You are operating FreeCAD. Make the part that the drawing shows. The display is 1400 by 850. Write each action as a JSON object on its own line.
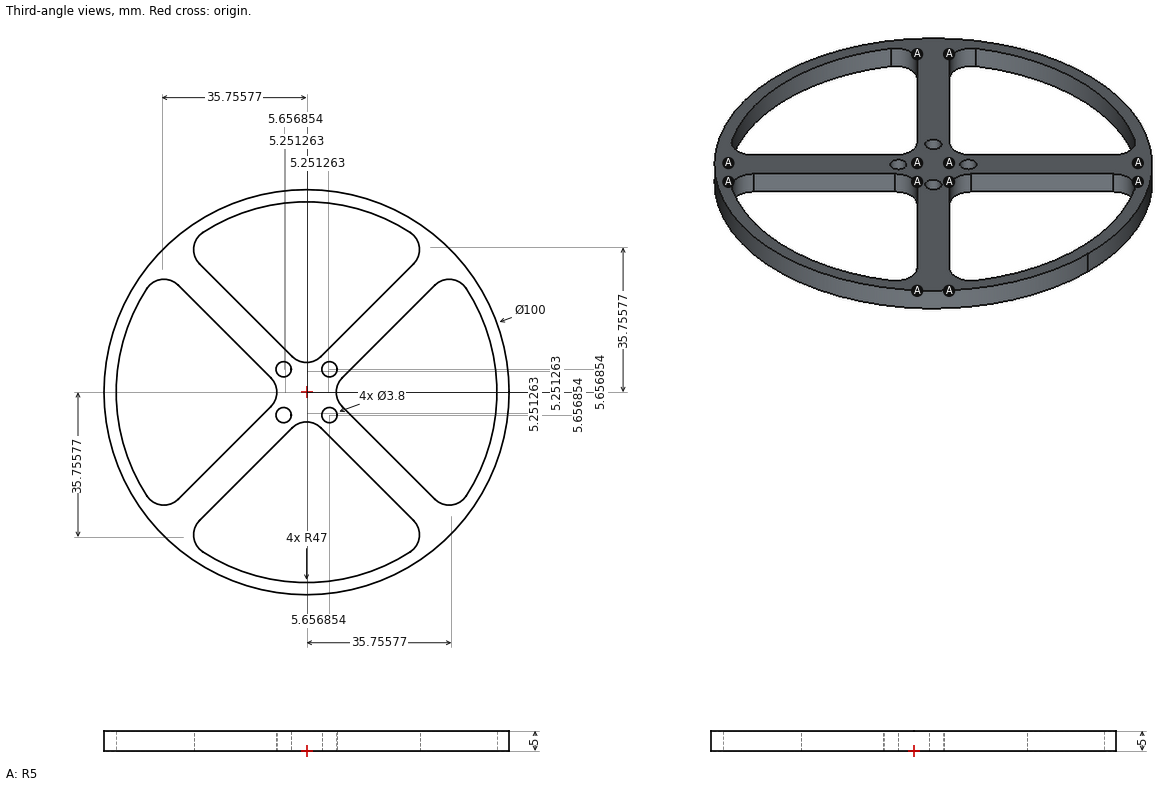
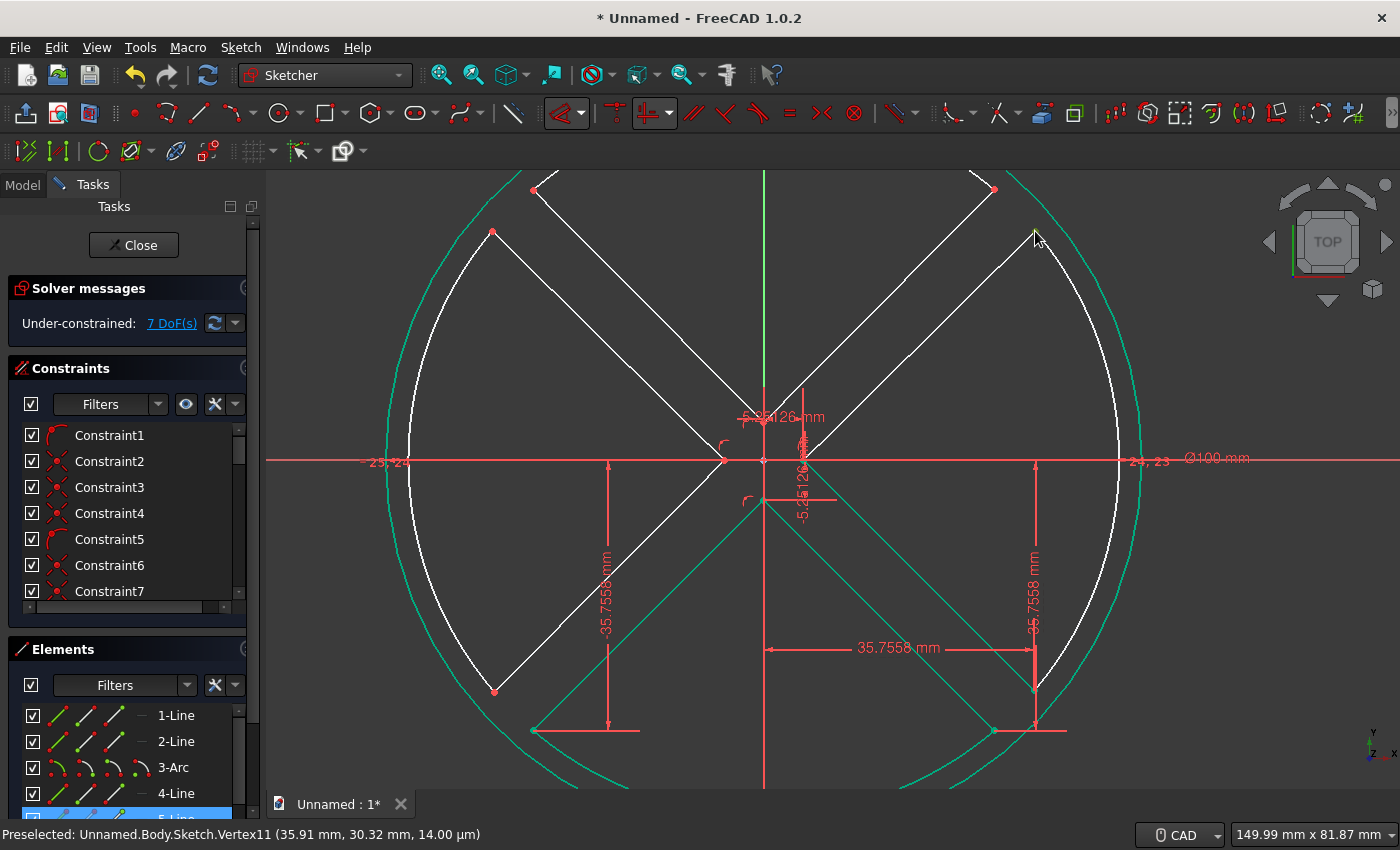
{"action": "key", "text": "l"}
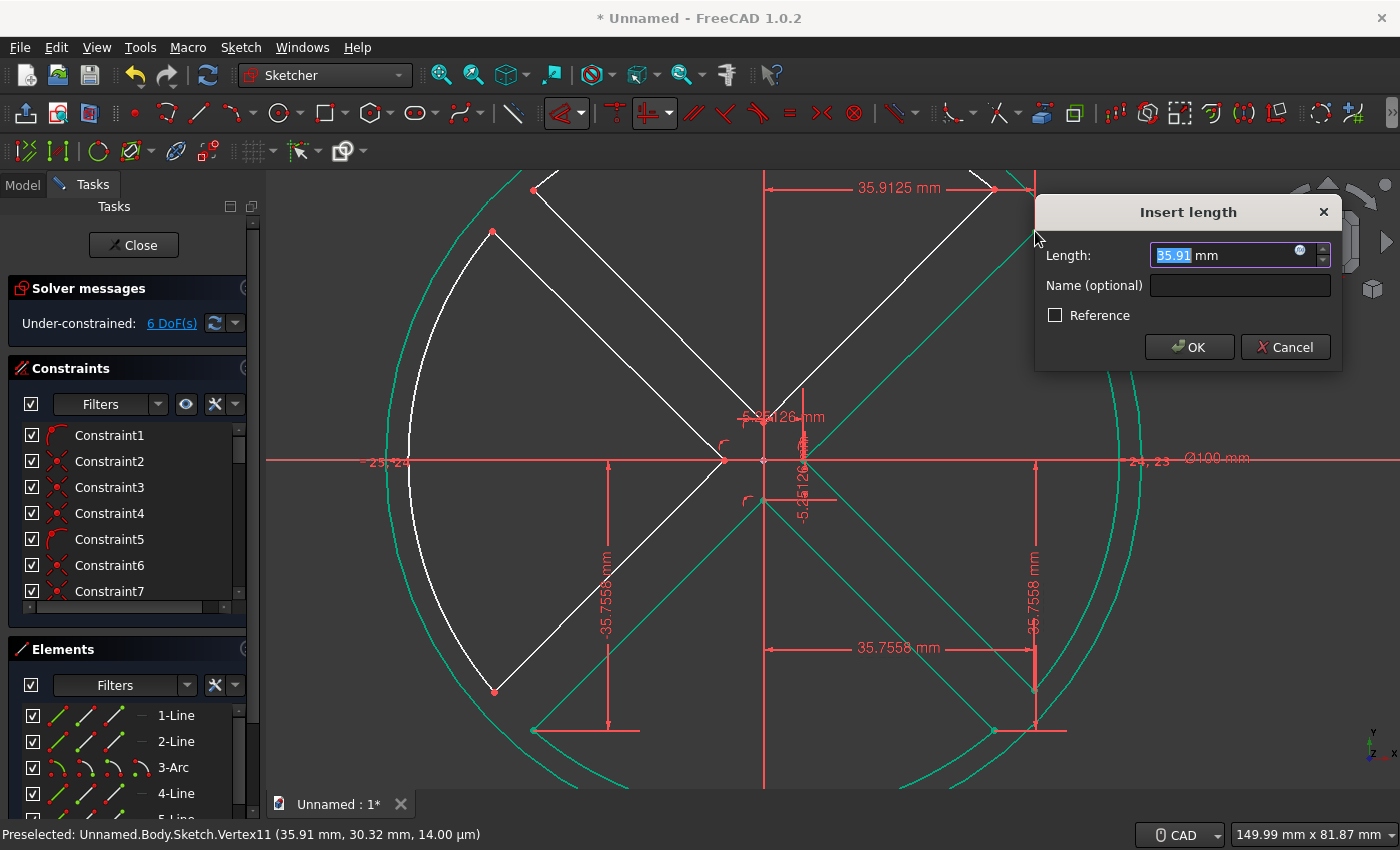
{"action": "type", "text": "35.75577"}
{"action": "key", "text": "Return"}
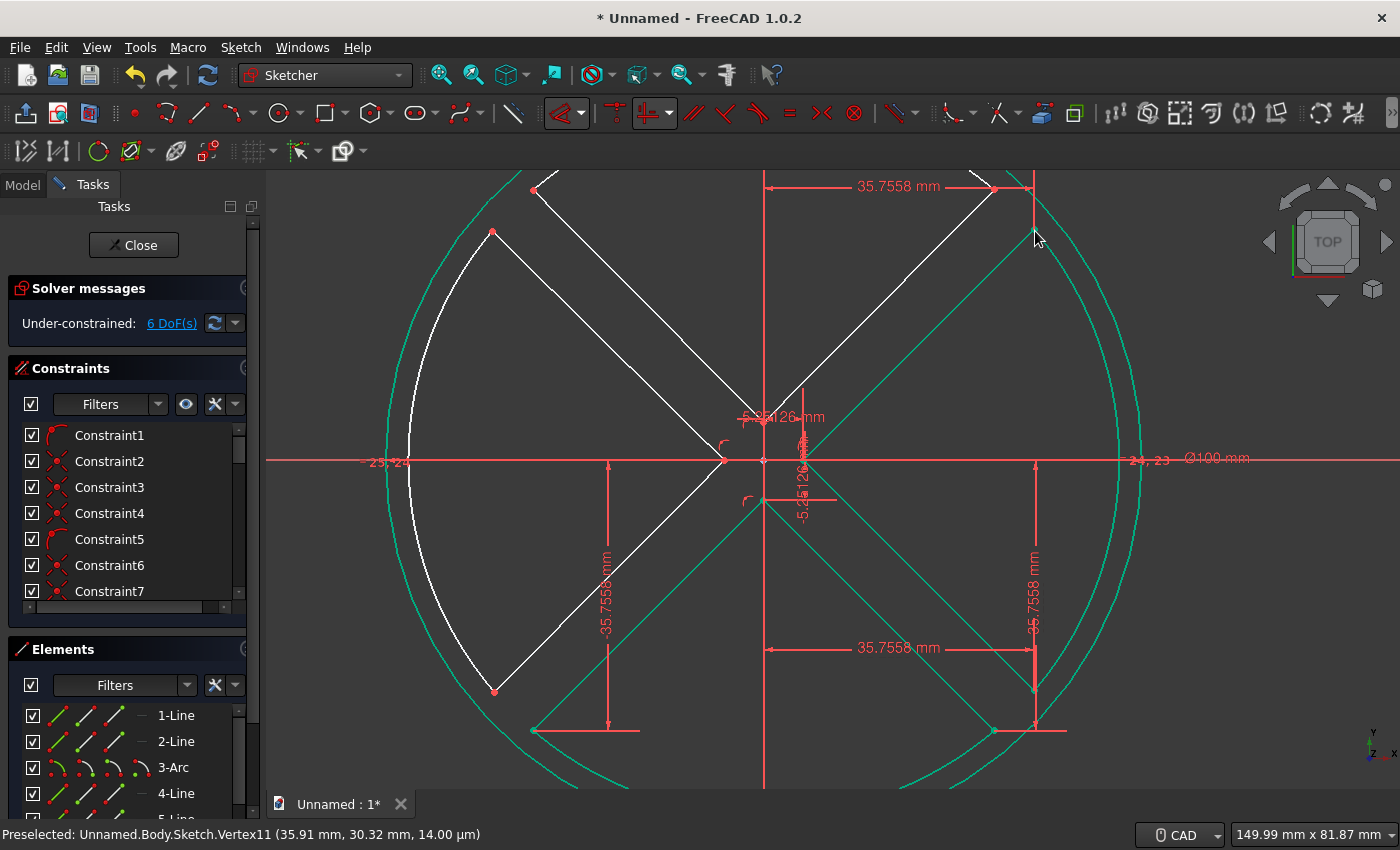
{"action": "left_click", "coordinate": [492, 231]}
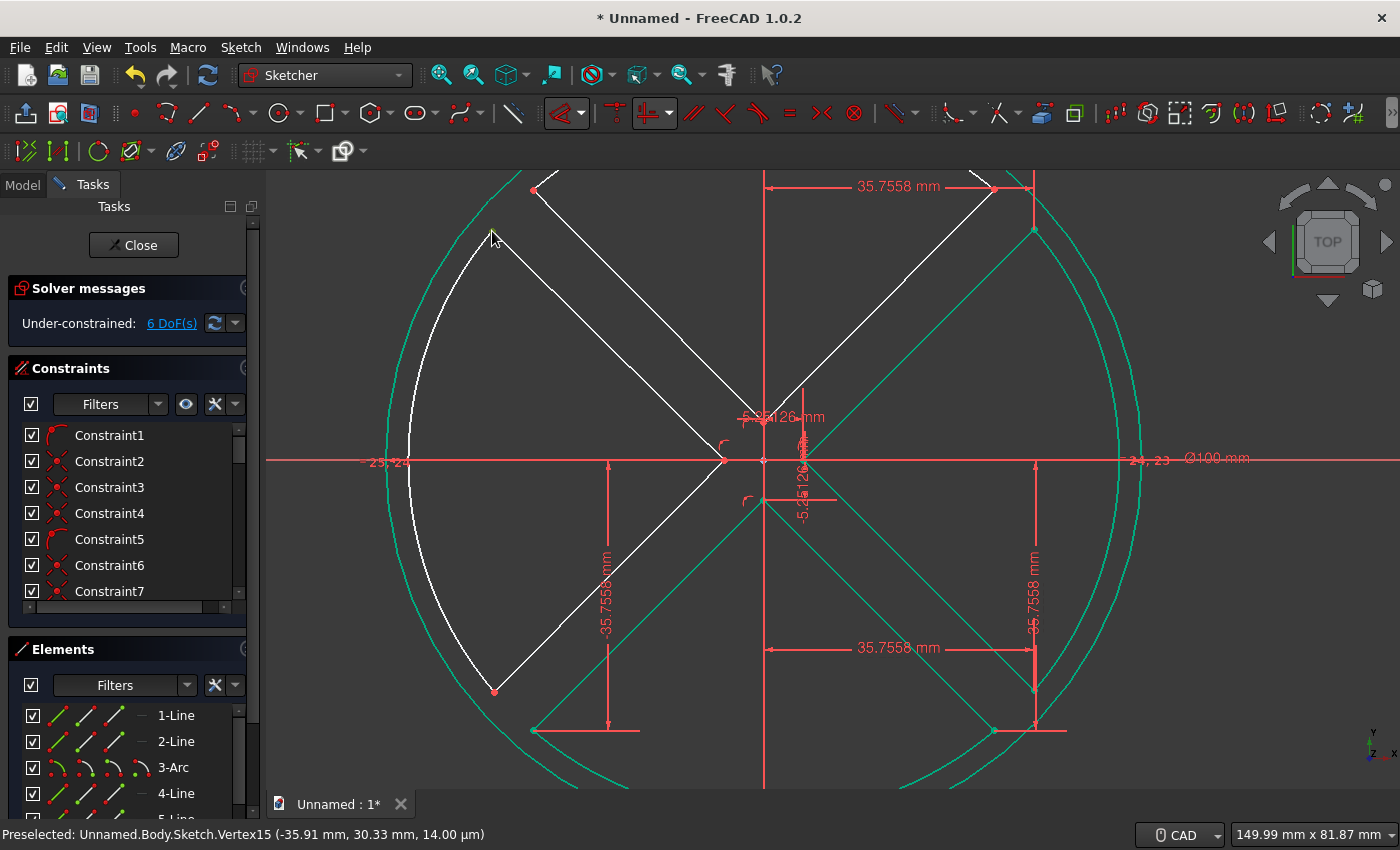
{"action": "key", "text": "l"}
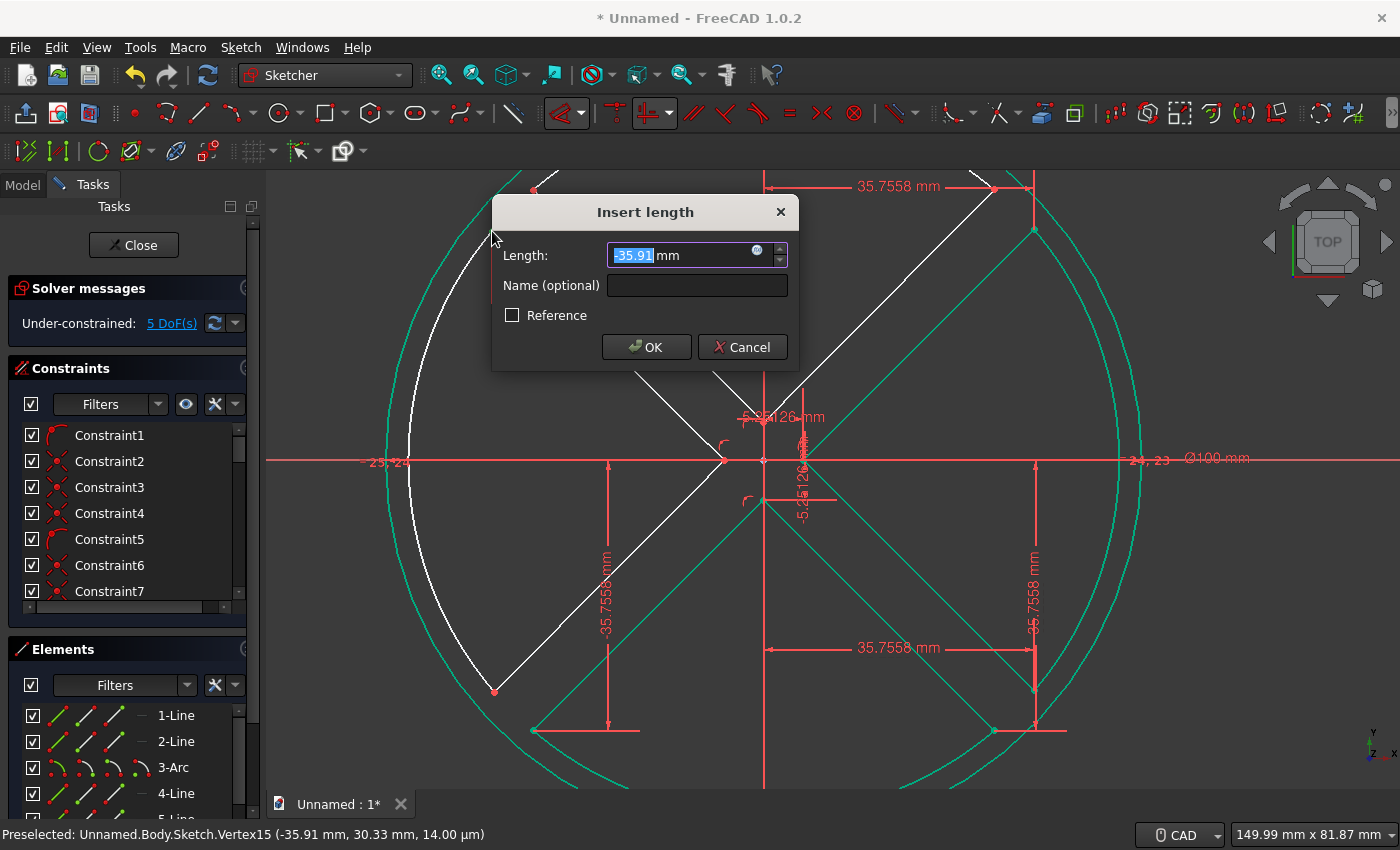
{"action": "type", "text": "-35.75577"}
{"action": "key", "text": "Return"}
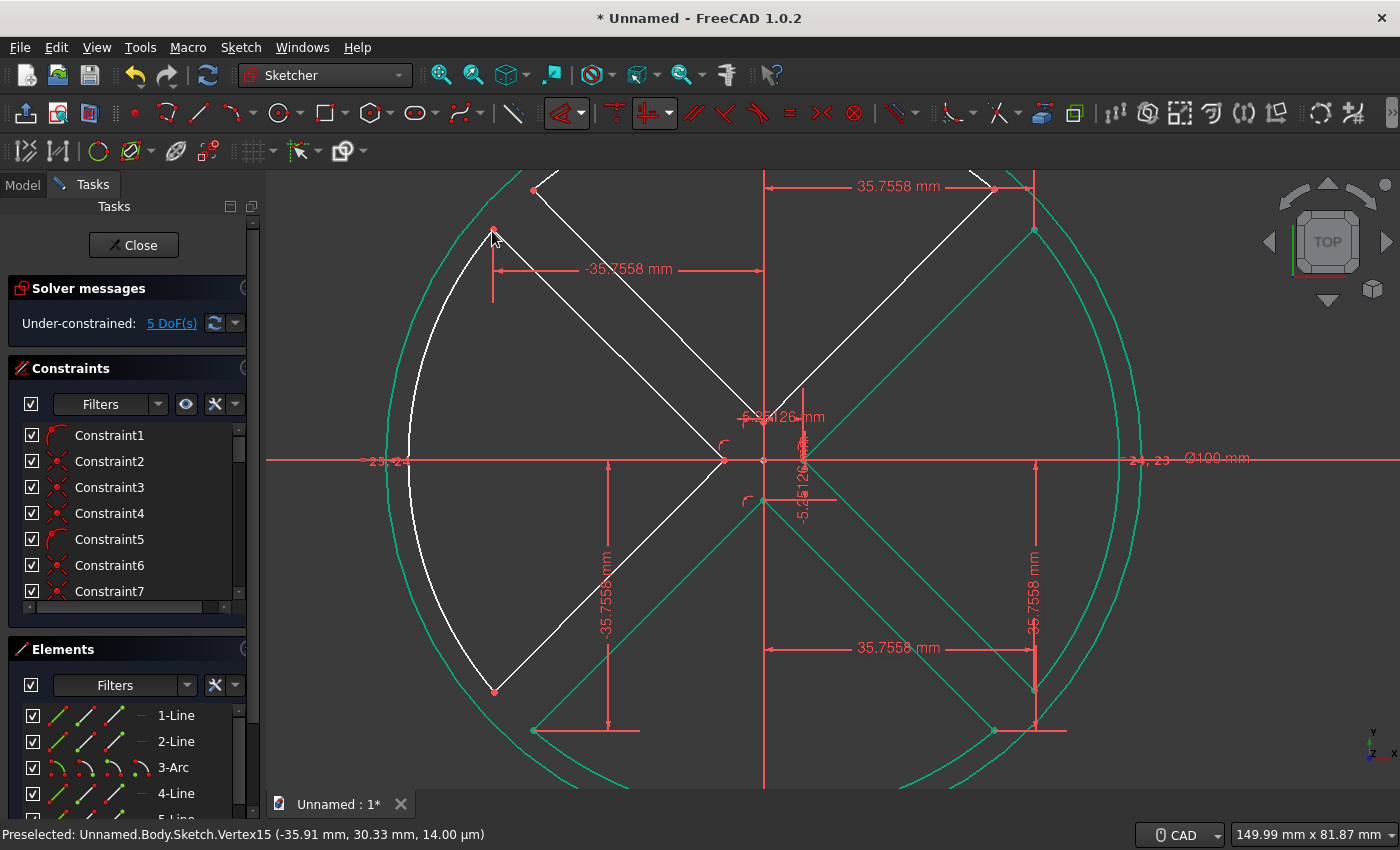
{"action": "left_click", "coordinate": [725, 460]}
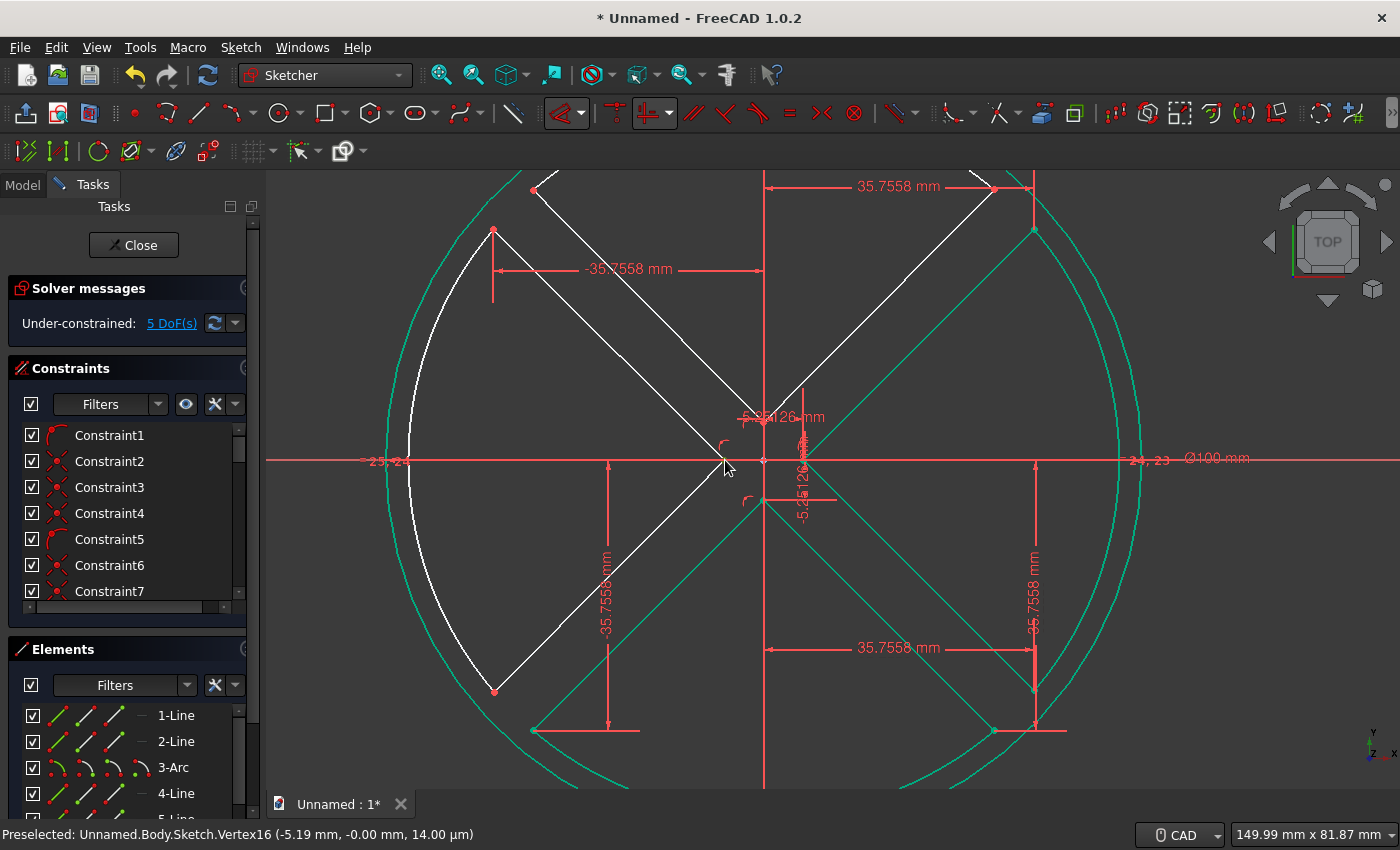
{"action": "key", "text": "l"}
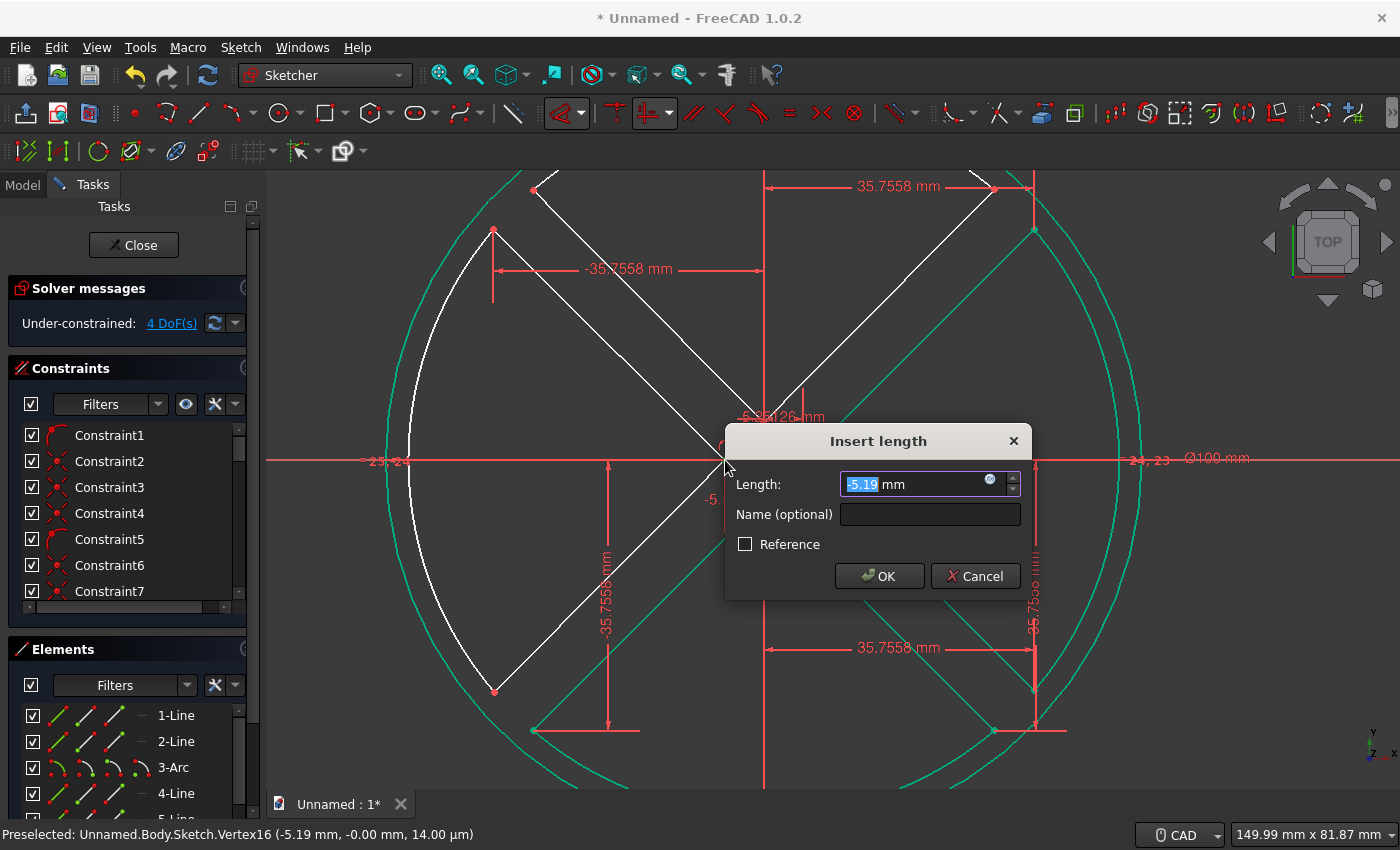
{"action": "type", "text": "-5.251263"}
{"action": "key", "text": "Return"}